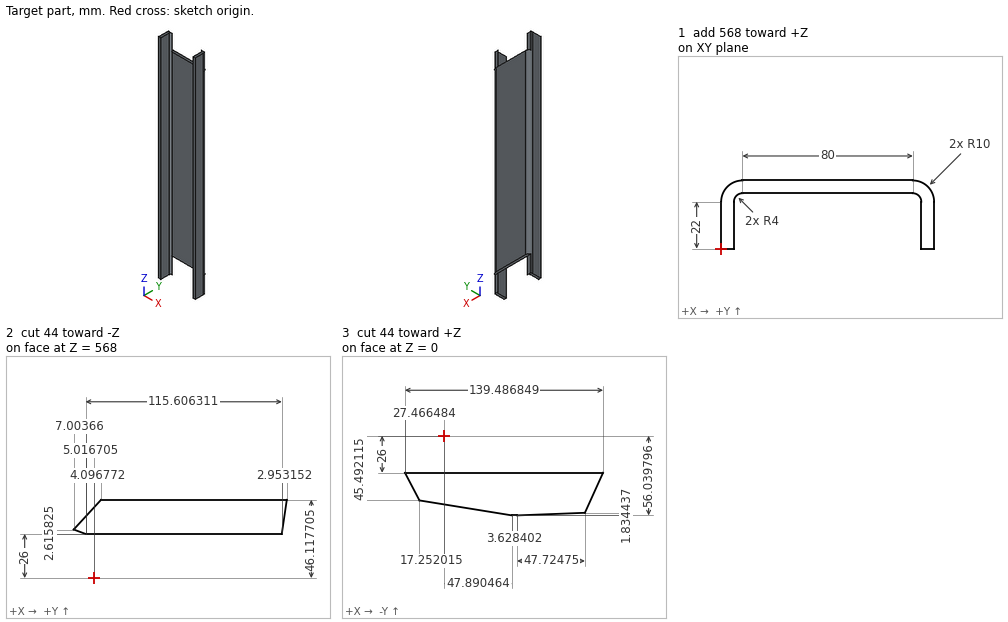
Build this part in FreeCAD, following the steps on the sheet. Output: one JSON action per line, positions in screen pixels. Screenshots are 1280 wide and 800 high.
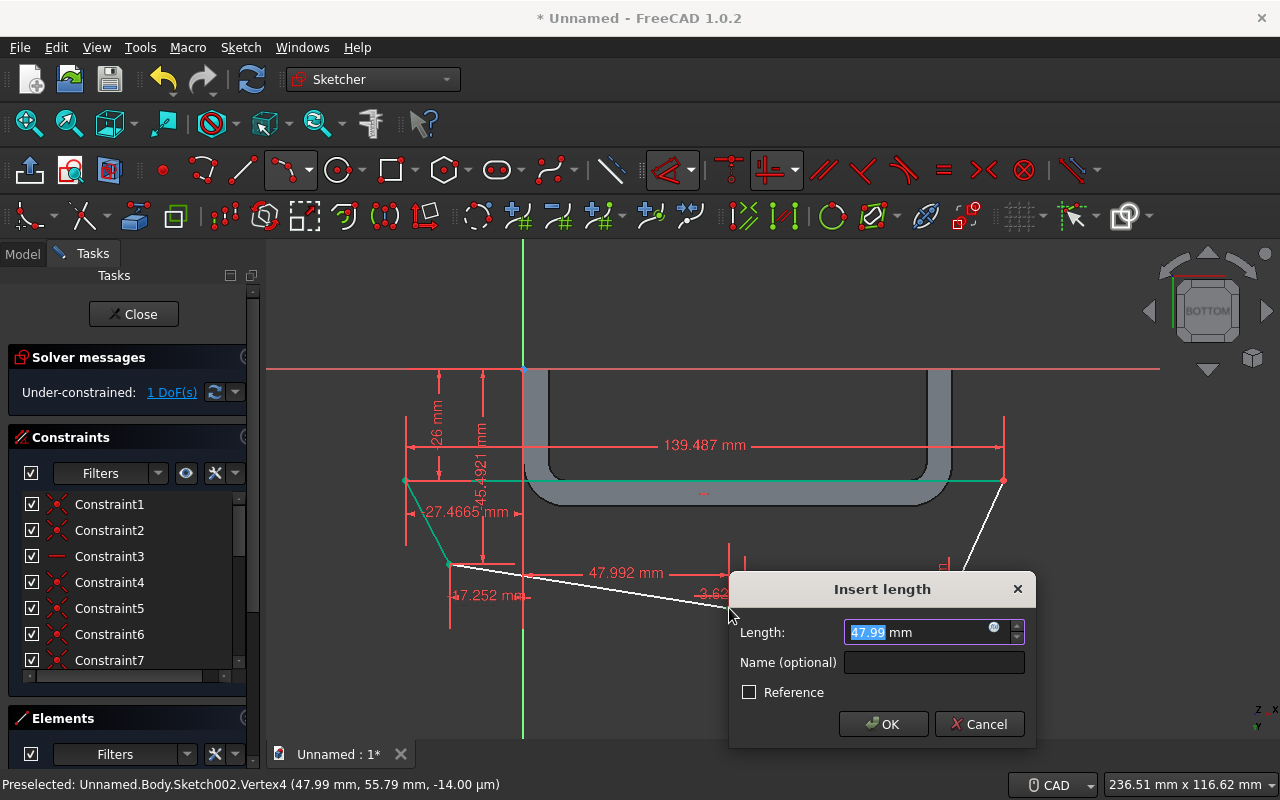
{"action": "type", "text": "47.890464"}
{"action": "key", "text": "Return"}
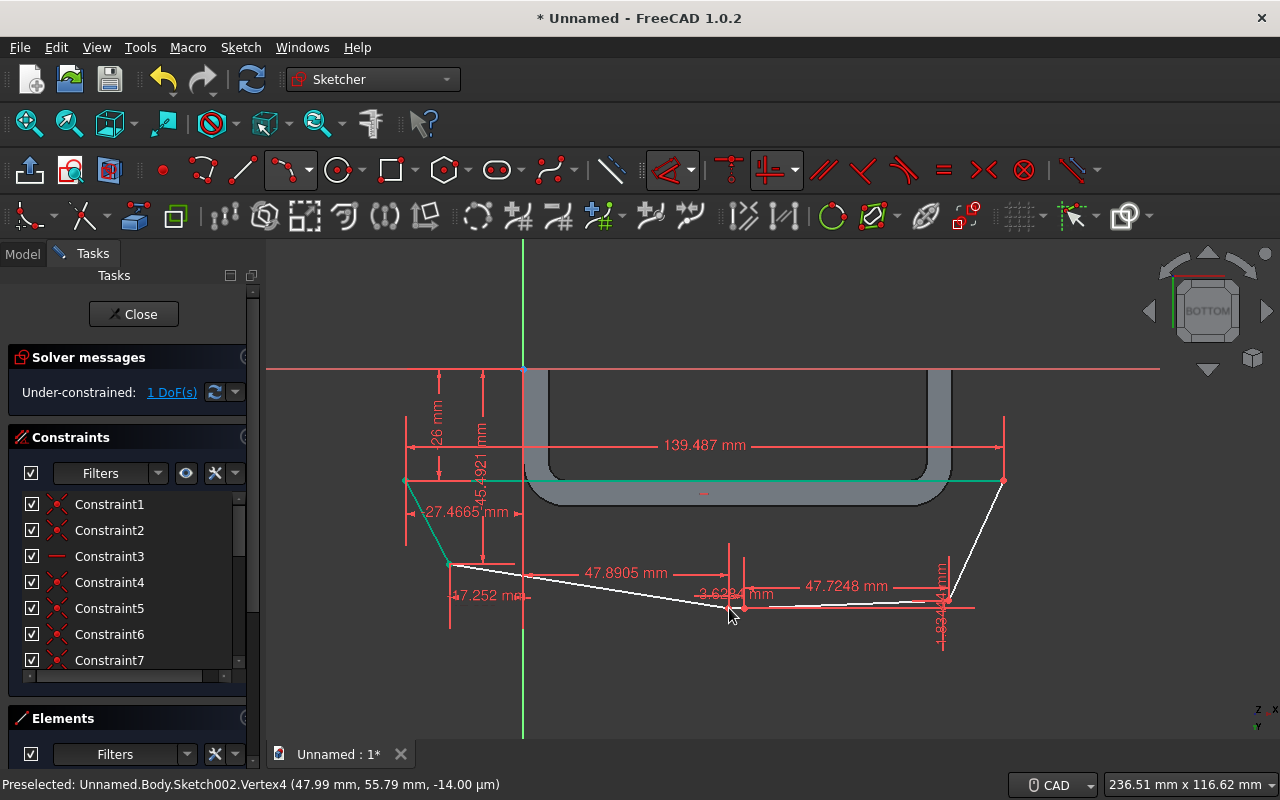
{"action": "left_click", "coordinate": [729, 608]}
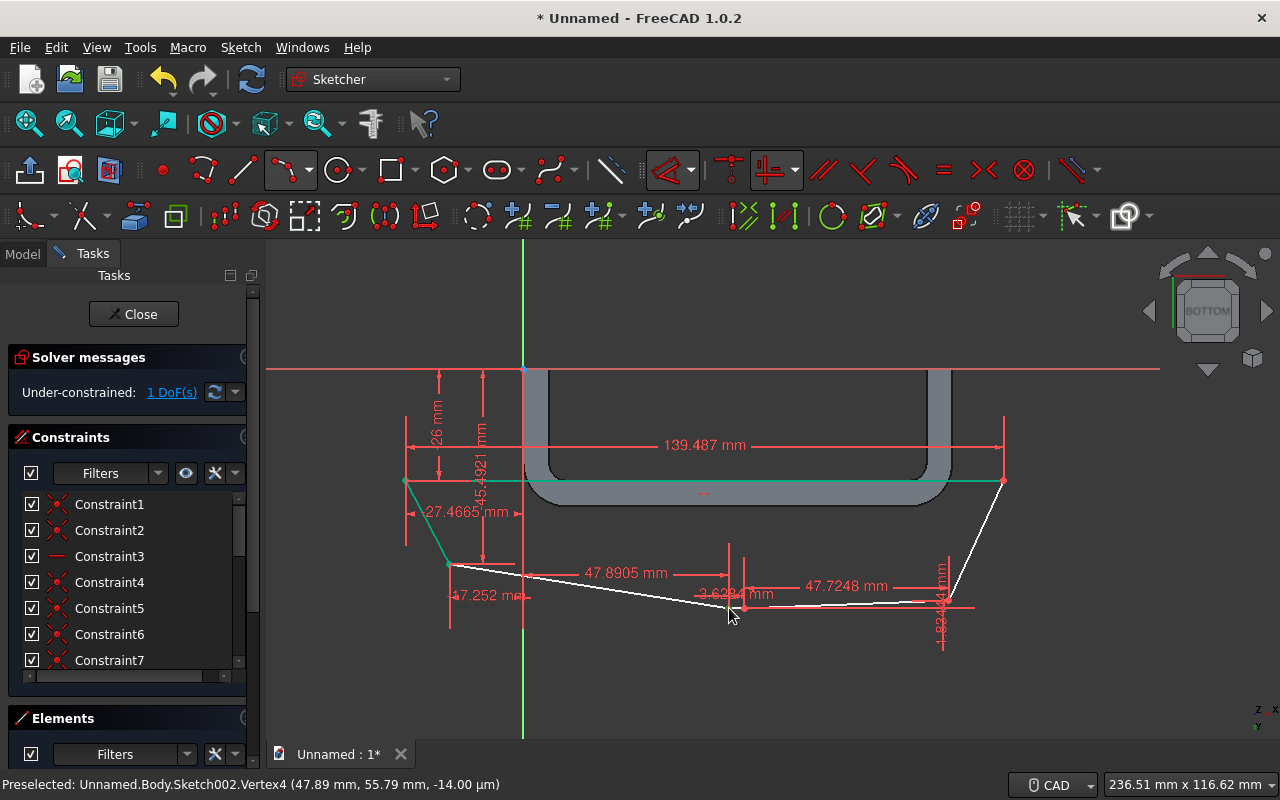
{"action": "key", "text": "i"}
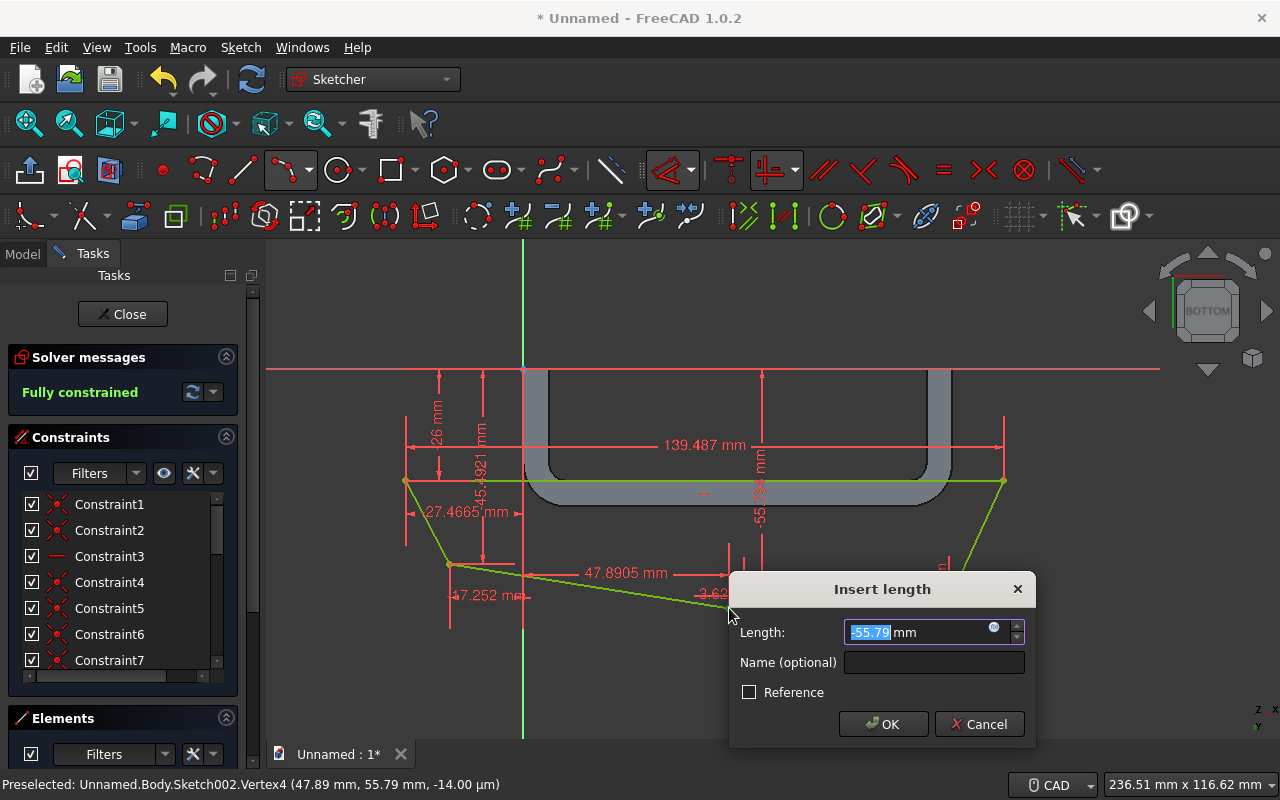
{"action": "type", "text": "-56.039796"}
{"action": "key", "text": "Return"}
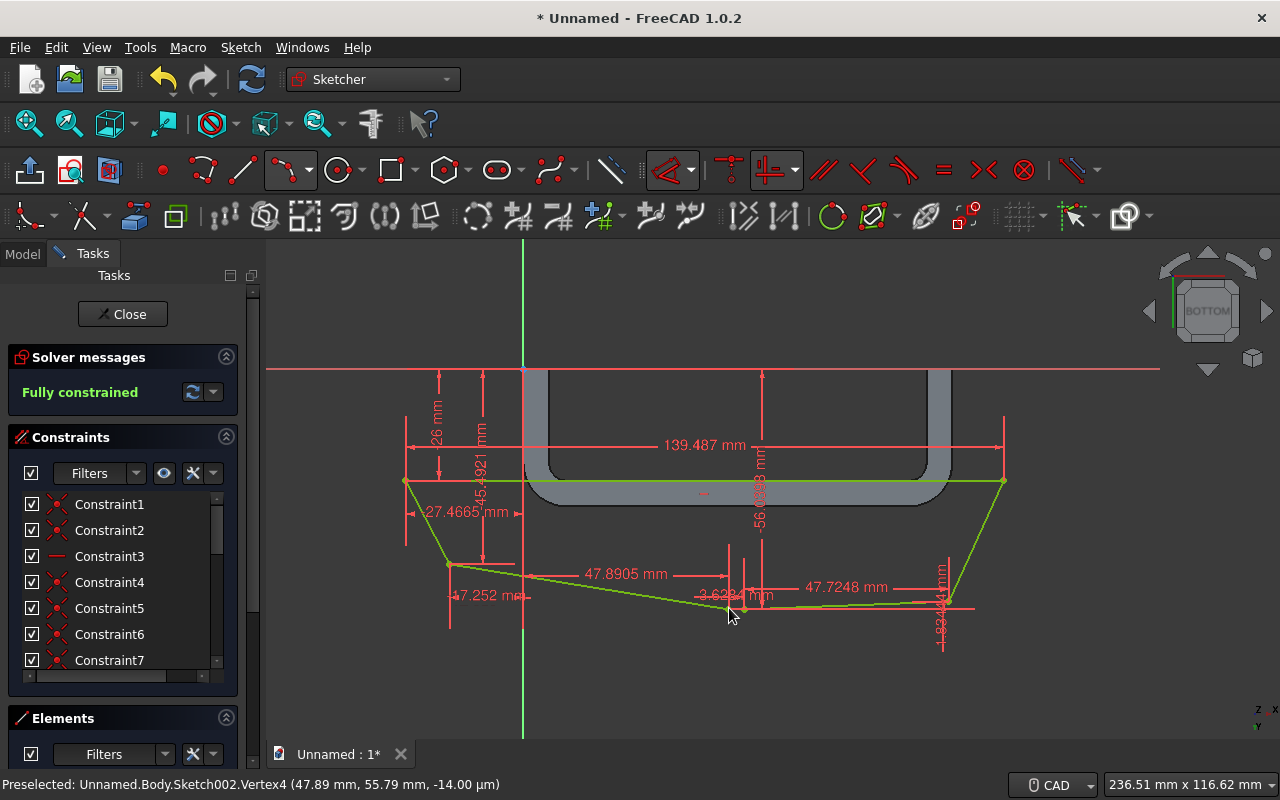
{"action": "left_click", "coordinate": [123, 314]}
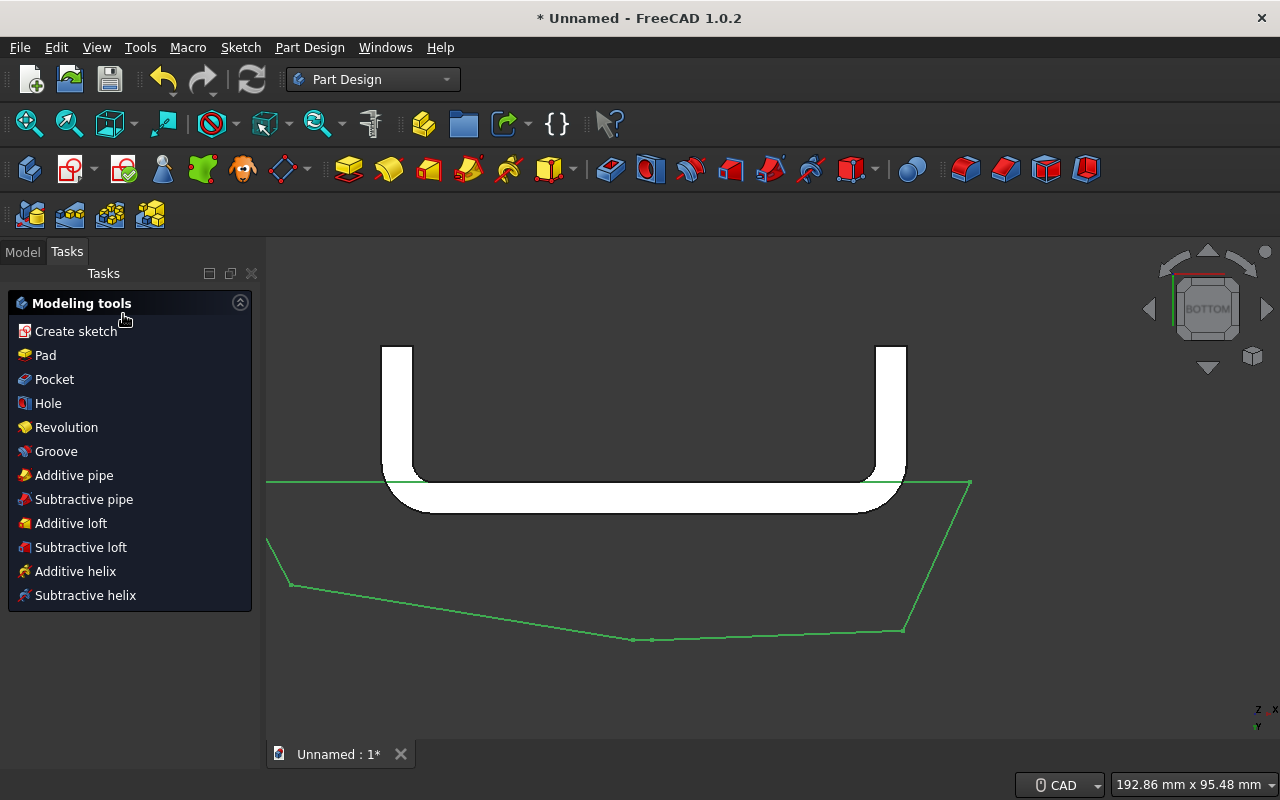
{"action": "left_click", "coordinate": [612, 170]}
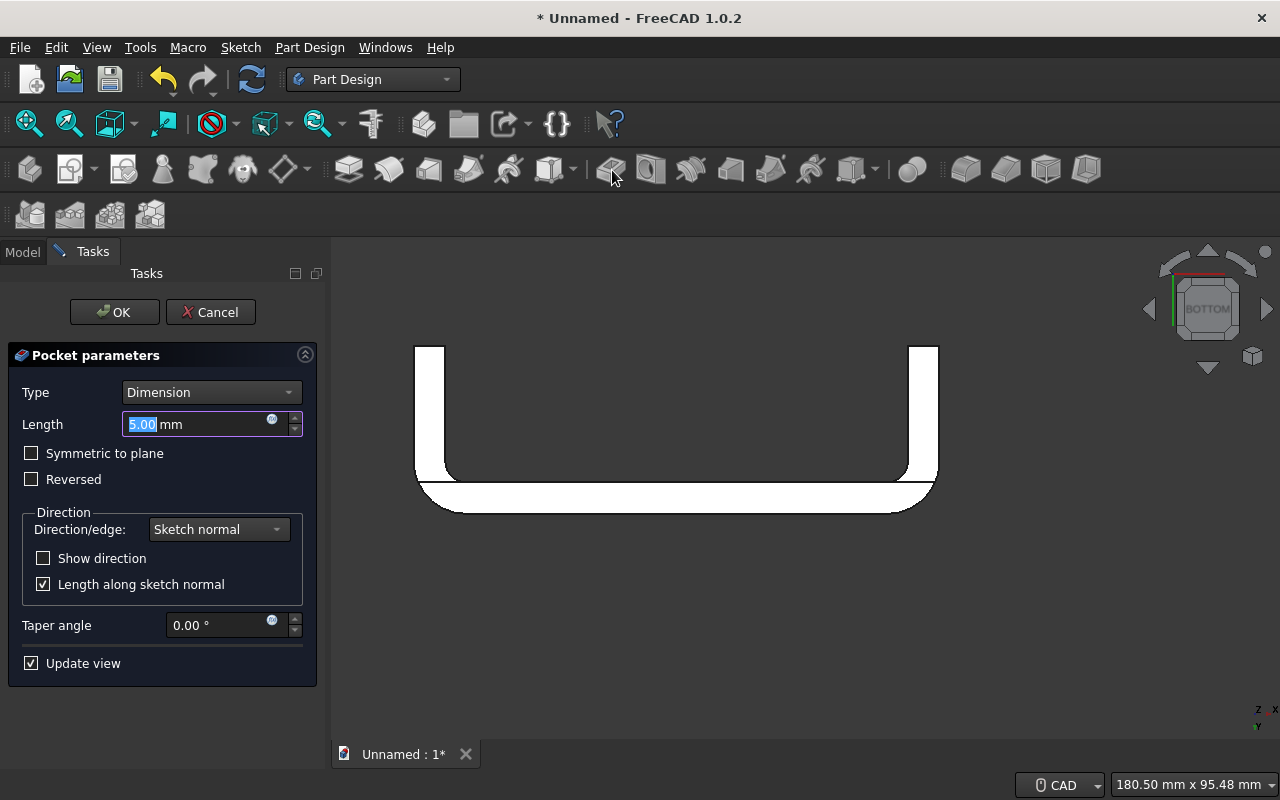
{"action": "type", "text": "44"}
{"action": "key", "text": "Tab"}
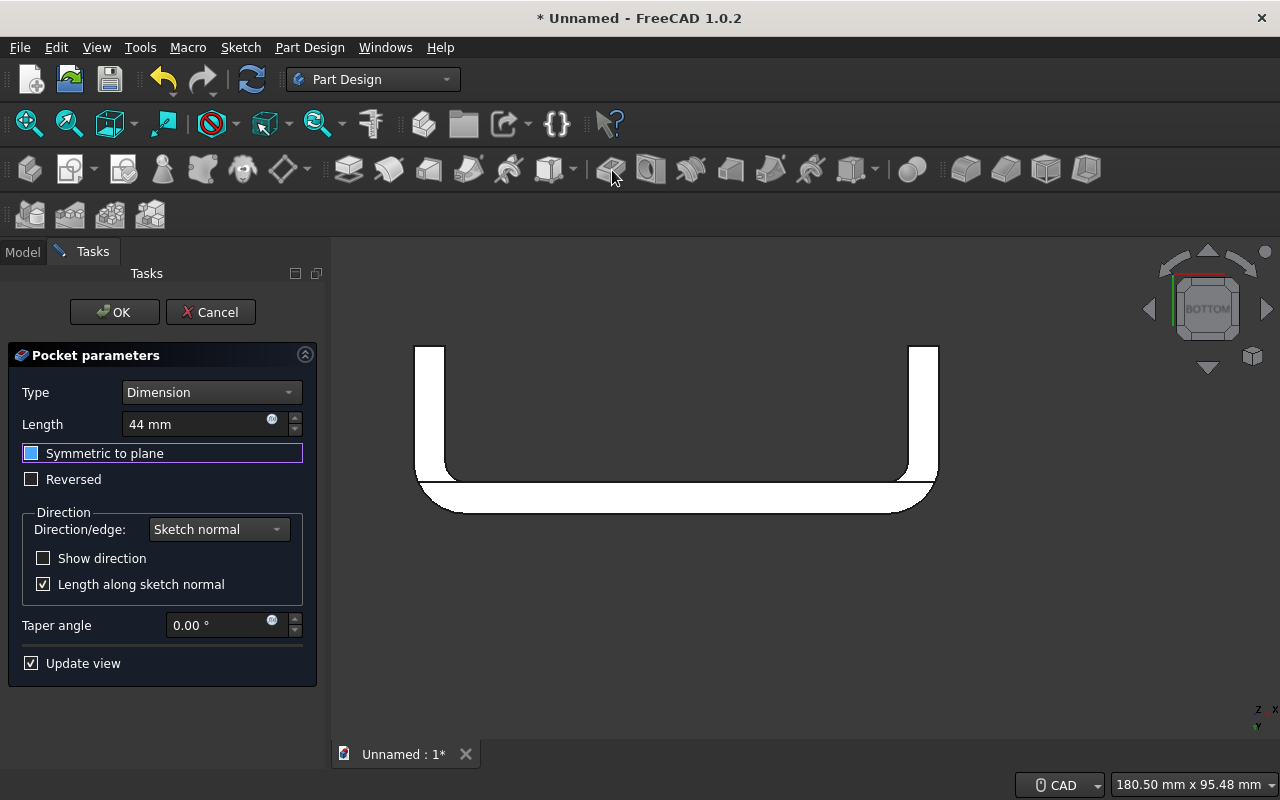
{"action": "left_click", "coordinate": [115, 312]}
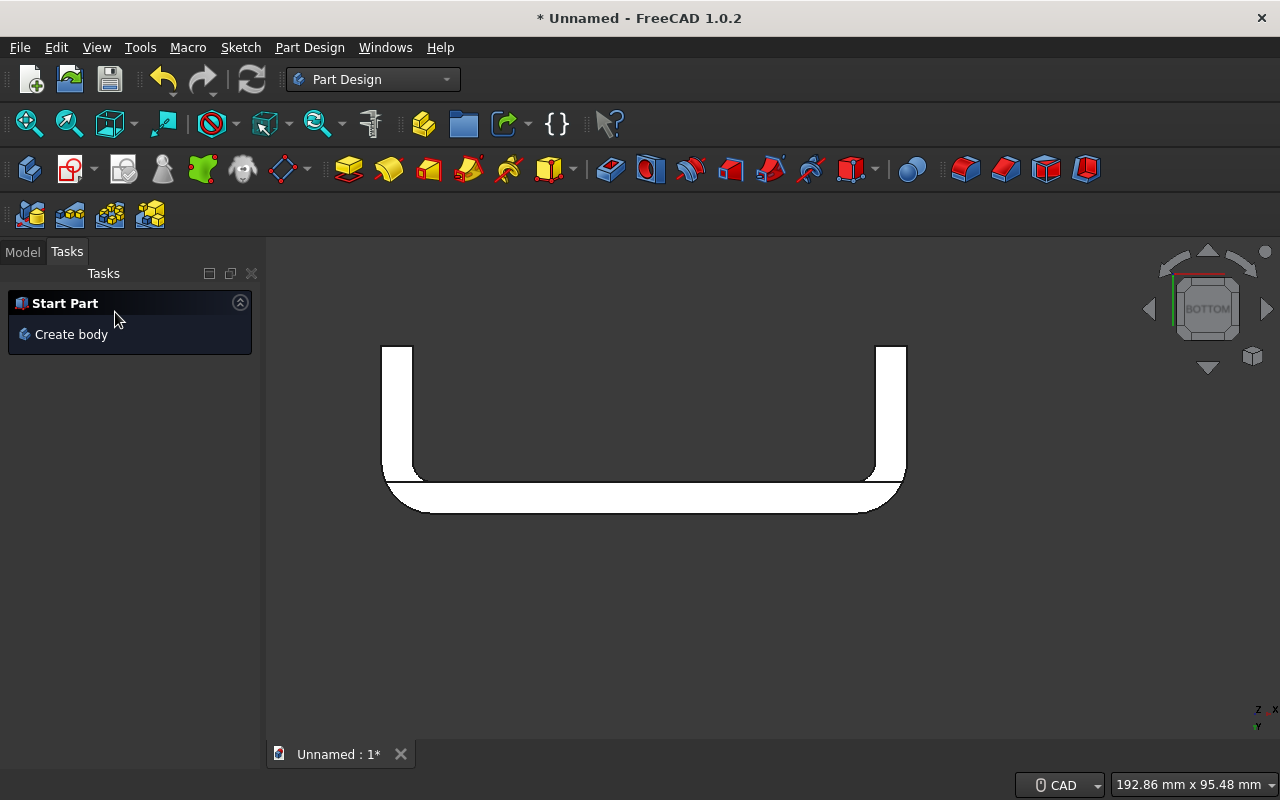
{"action": "key", "text": "0"}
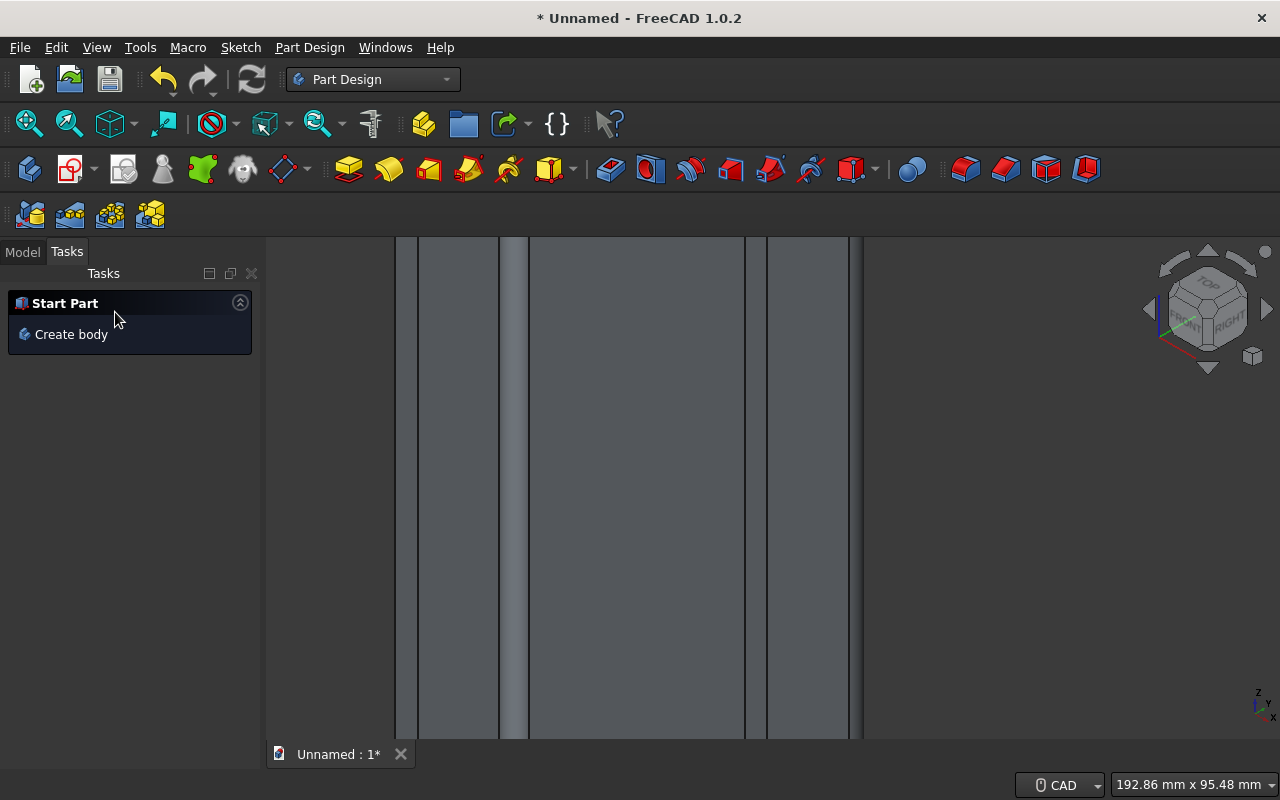
{"action": "left_click", "coordinate": [30, 124]}